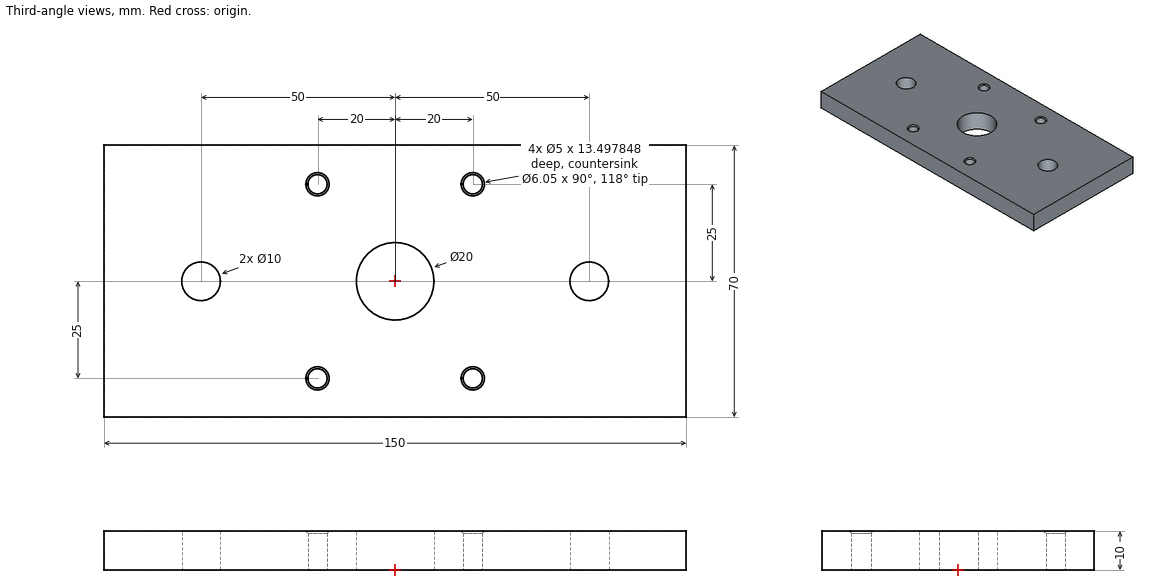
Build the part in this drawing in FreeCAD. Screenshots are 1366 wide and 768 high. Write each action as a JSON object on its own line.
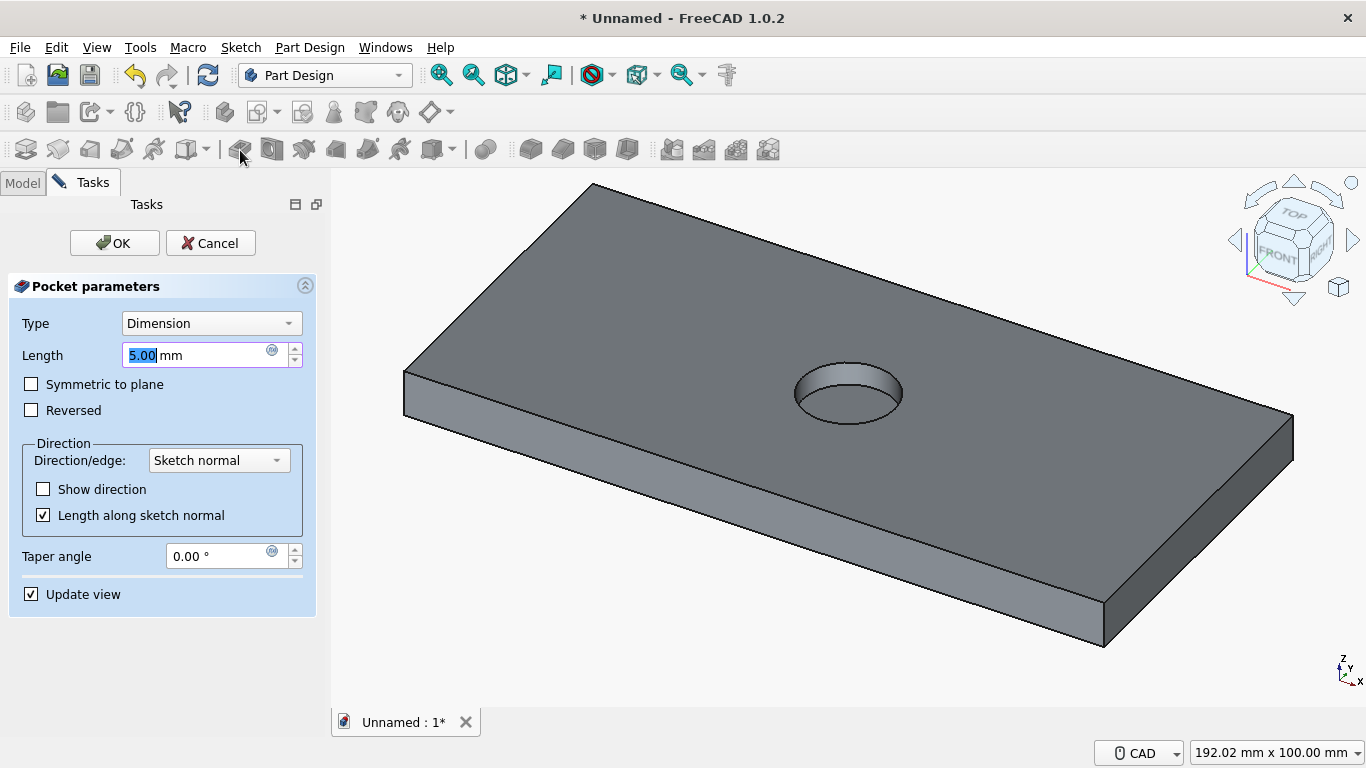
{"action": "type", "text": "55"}
{"action": "key", "text": "Tab"}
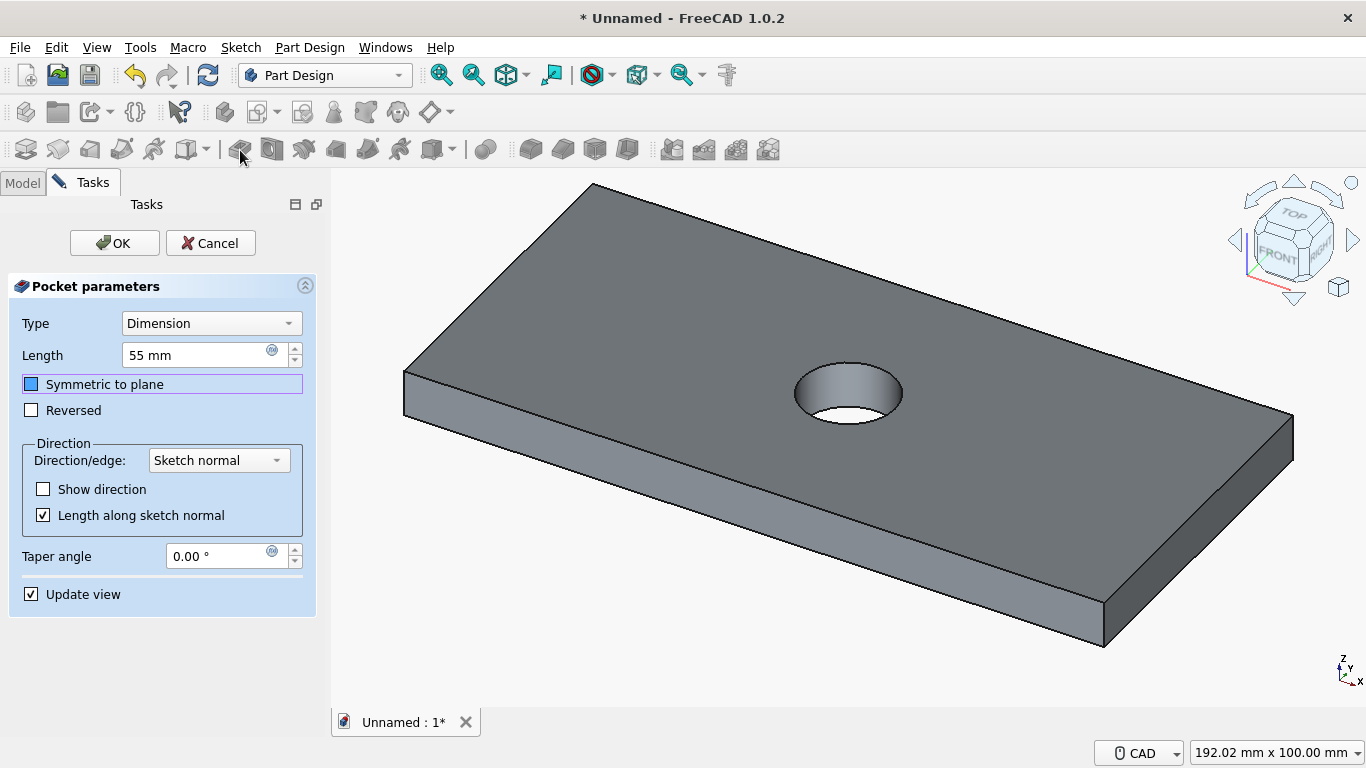
{"action": "left_click", "coordinate": [115, 243]}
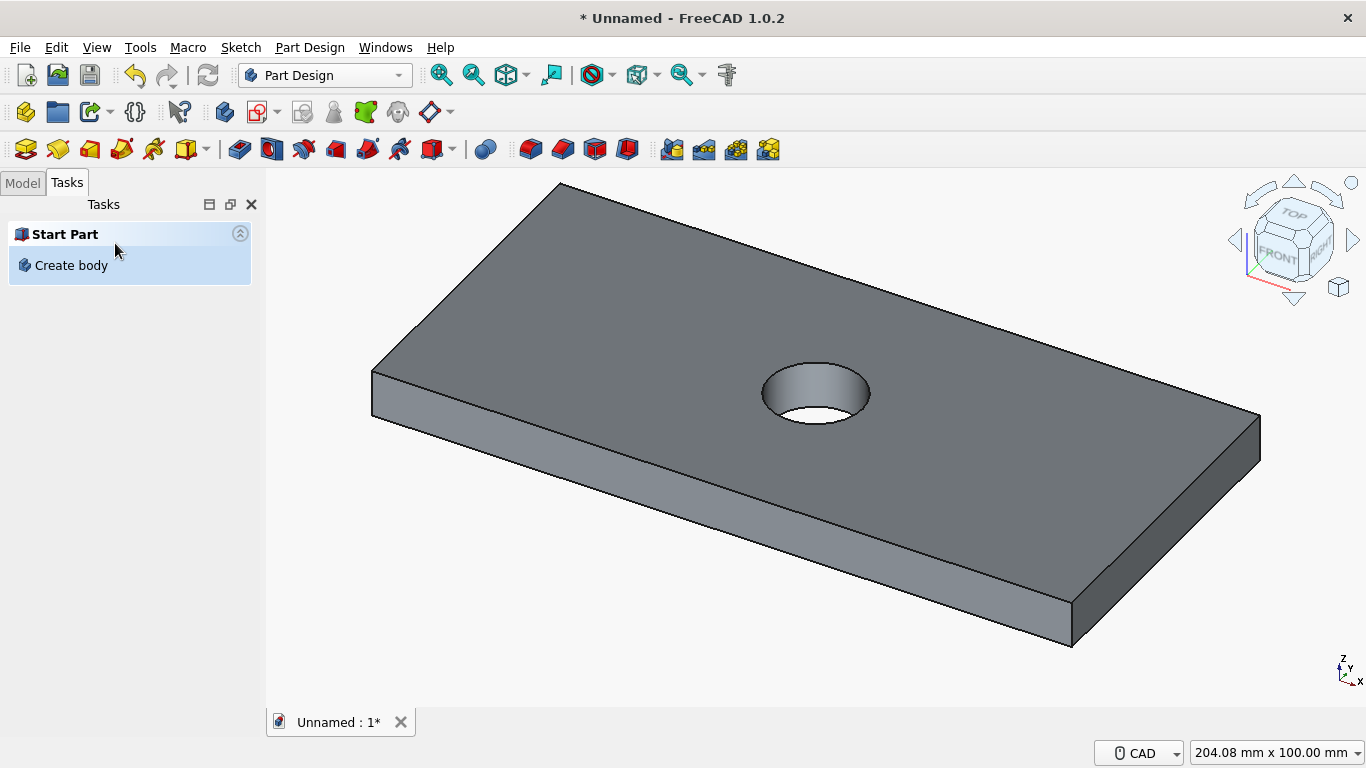
{"action": "left_click", "coordinate": [616, 326]}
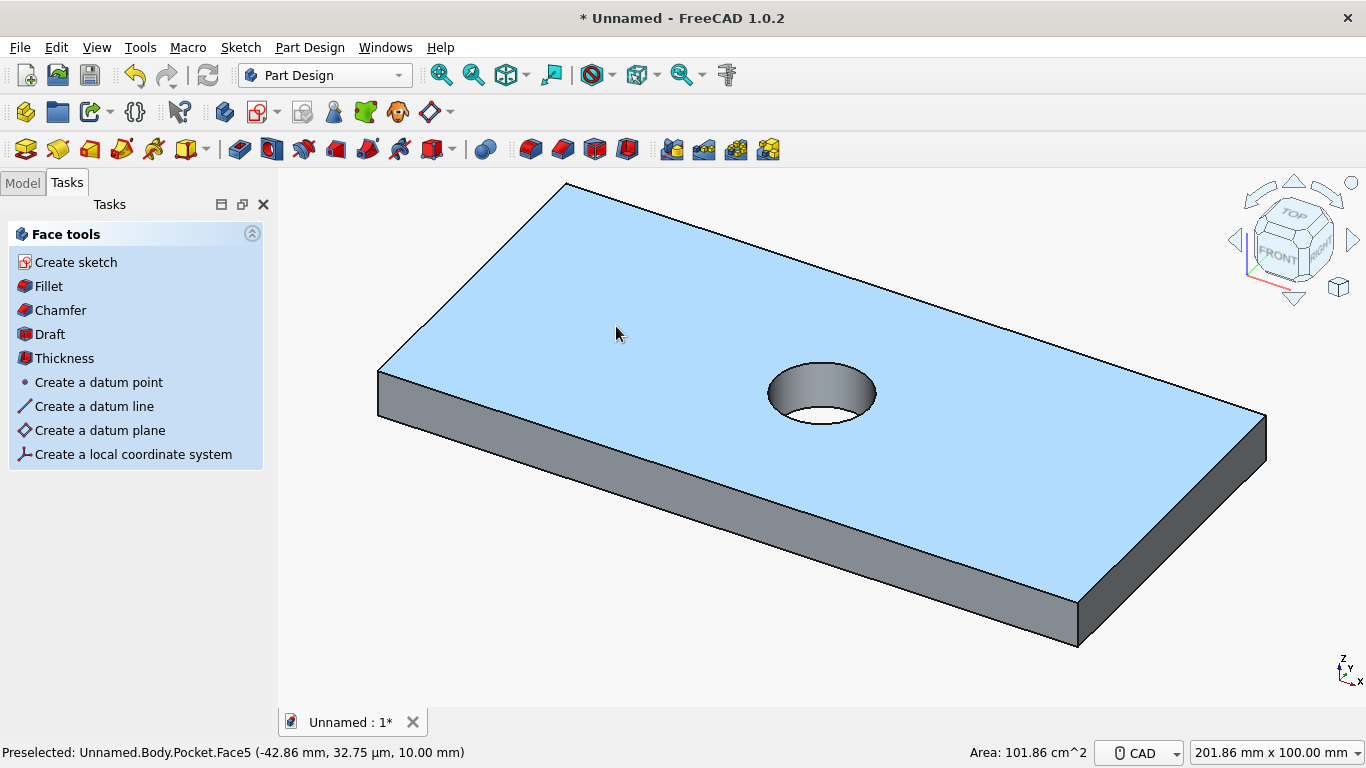
{"action": "left_click", "coordinate": [258, 112]}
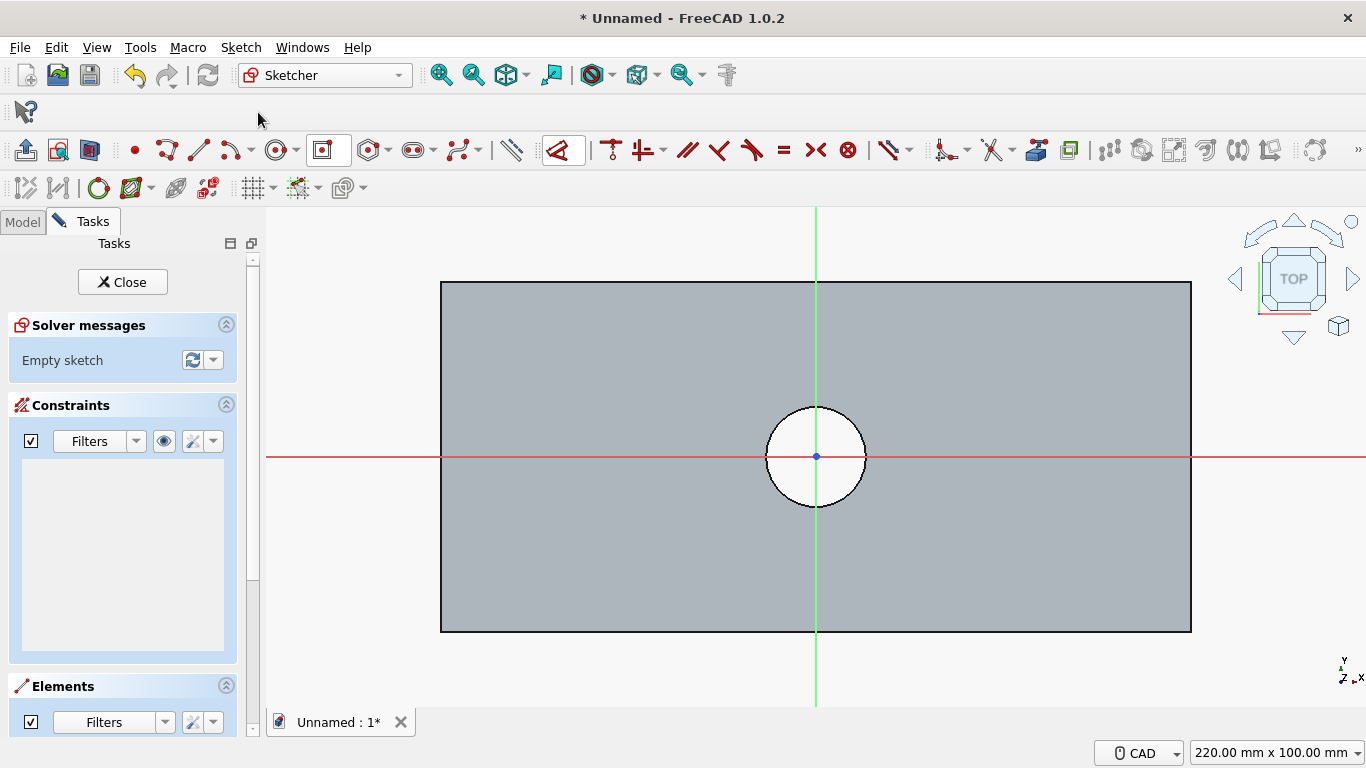
{"action": "left_click", "coordinate": [276, 150]}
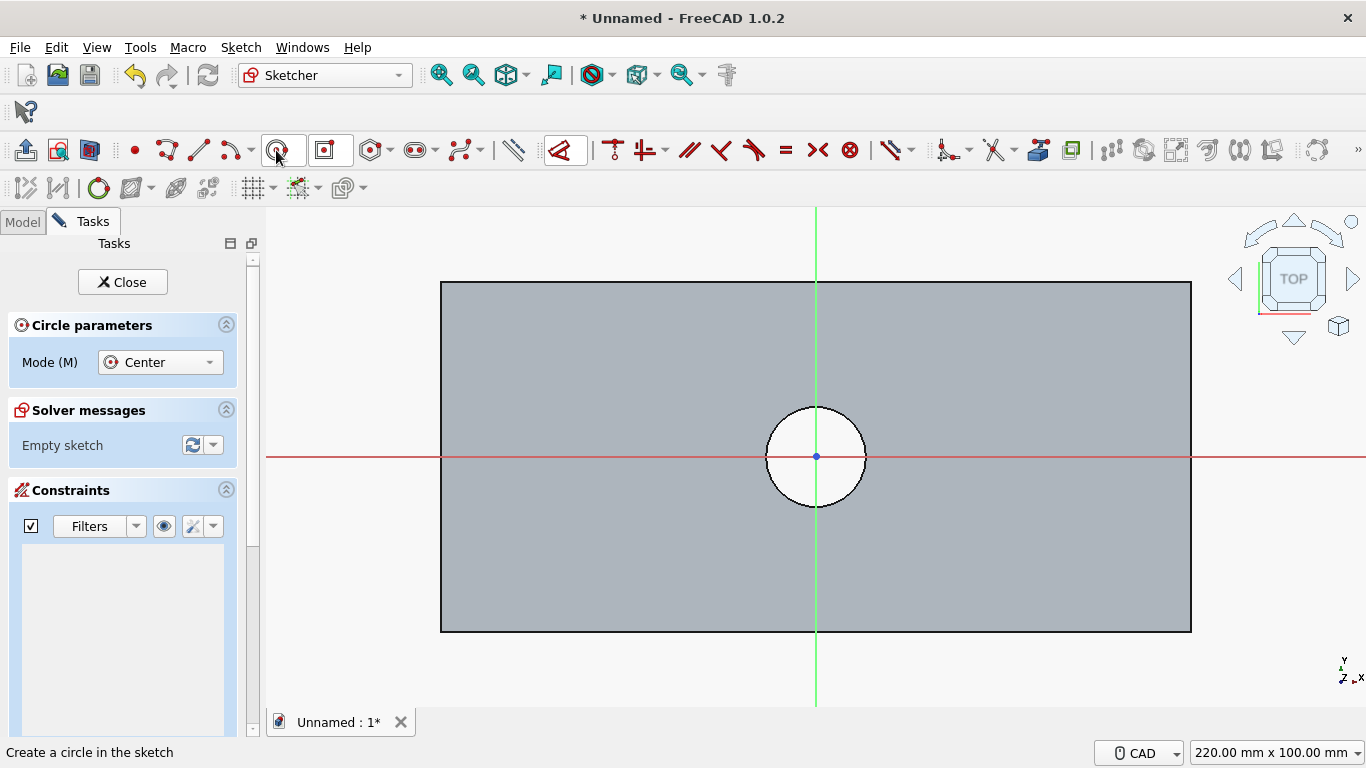
{"action": "left_click", "coordinate": [566, 457]}
{"action": "left_click", "coordinate": [584, 439]}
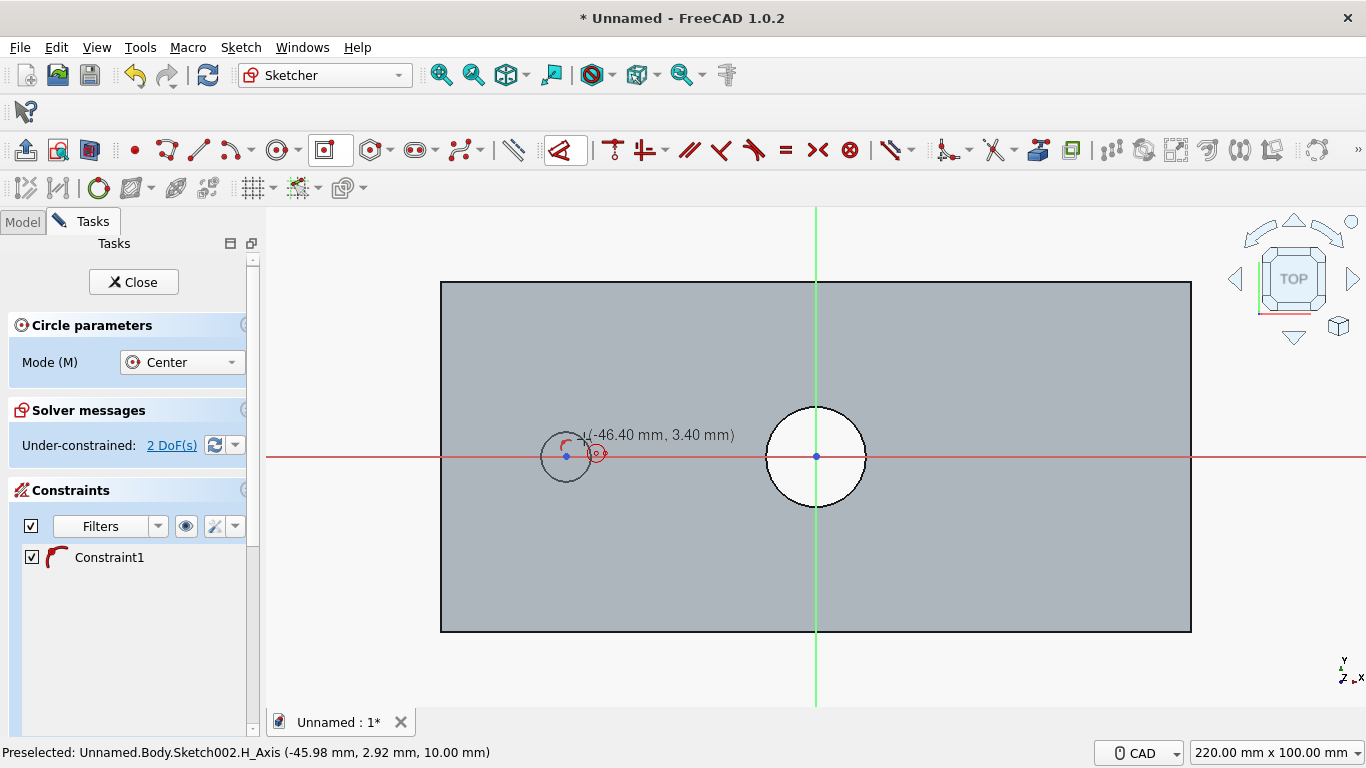
{"action": "left_click", "coordinate": [1066, 457]}
{"action": "left_click", "coordinate": [1084, 439]}
{"action": "key", "text": "Escape"}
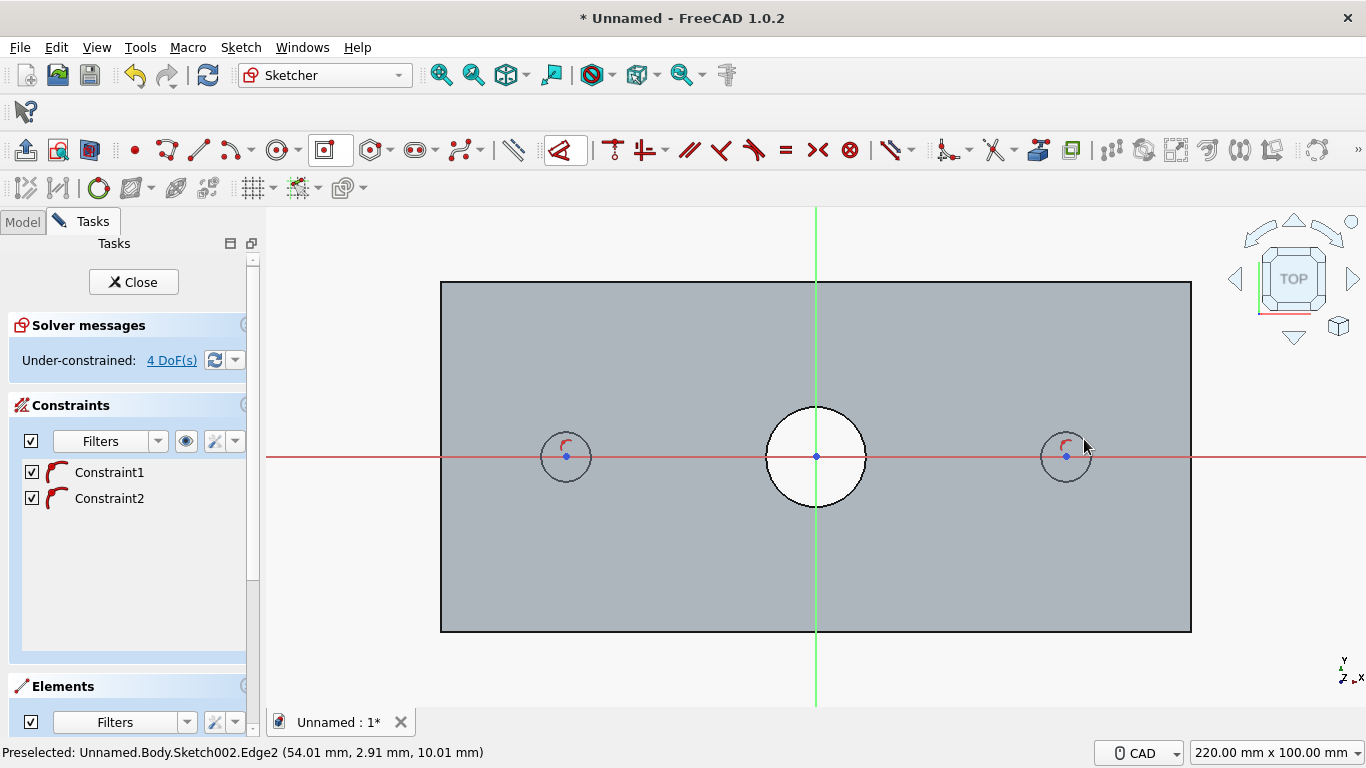
{"action": "left_click", "coordinate": [583, 439]}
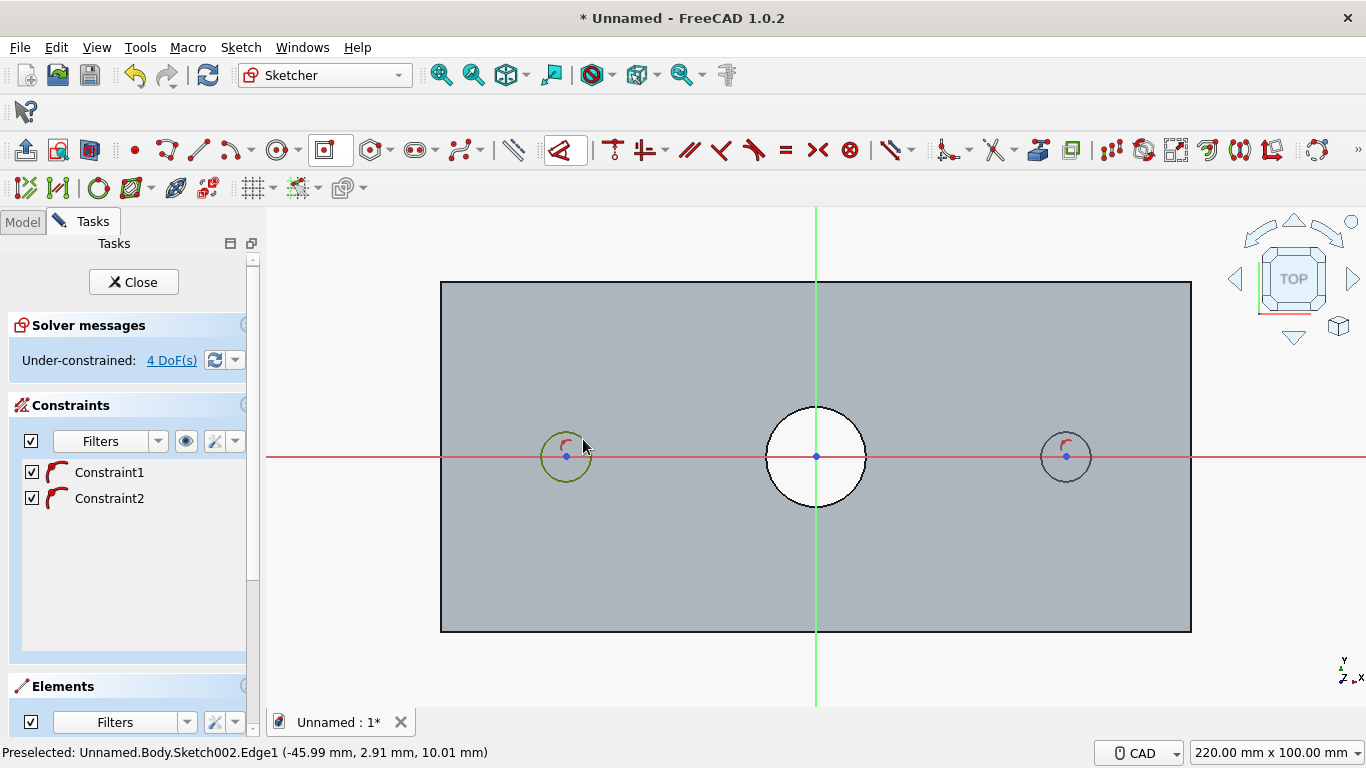
{"action": "left_click", "coordinate": [1083, 439]}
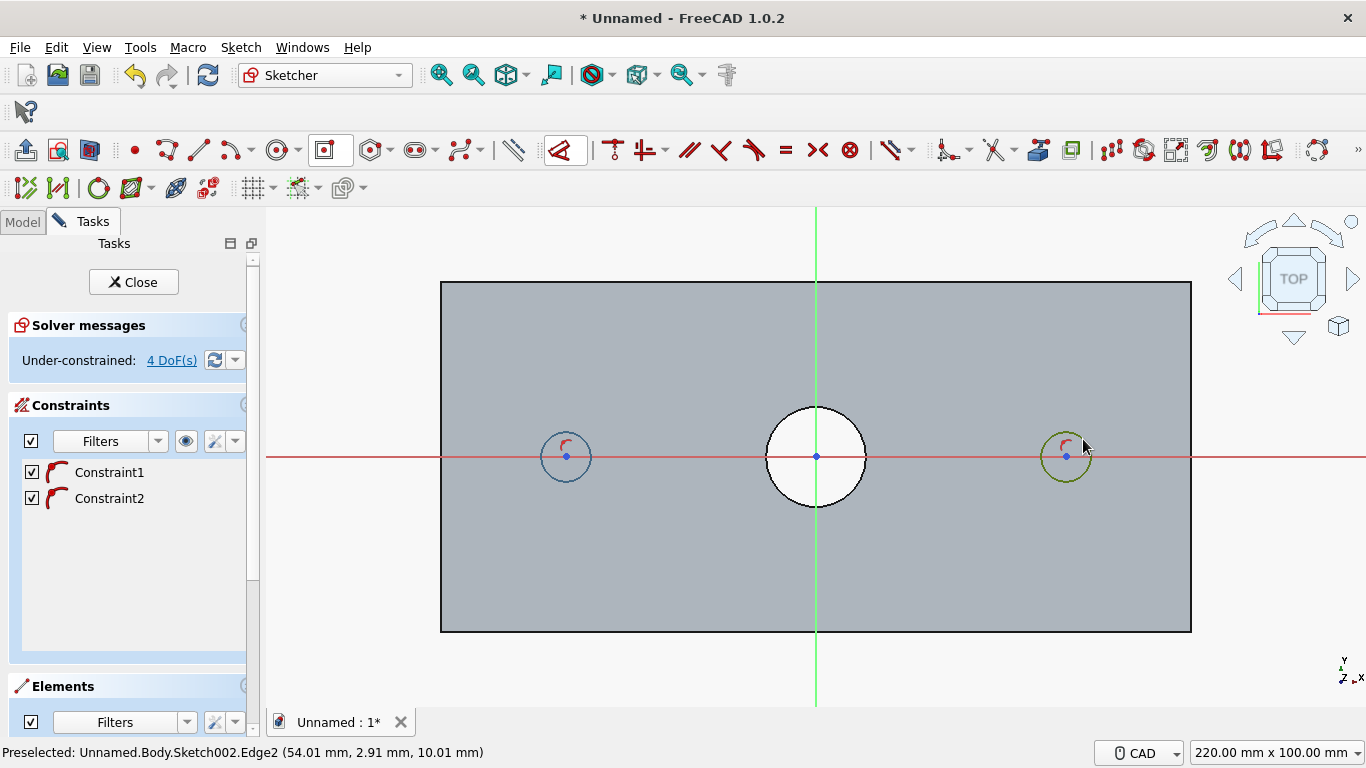
{"action": "left_click", "coordinate": [786, 150]}